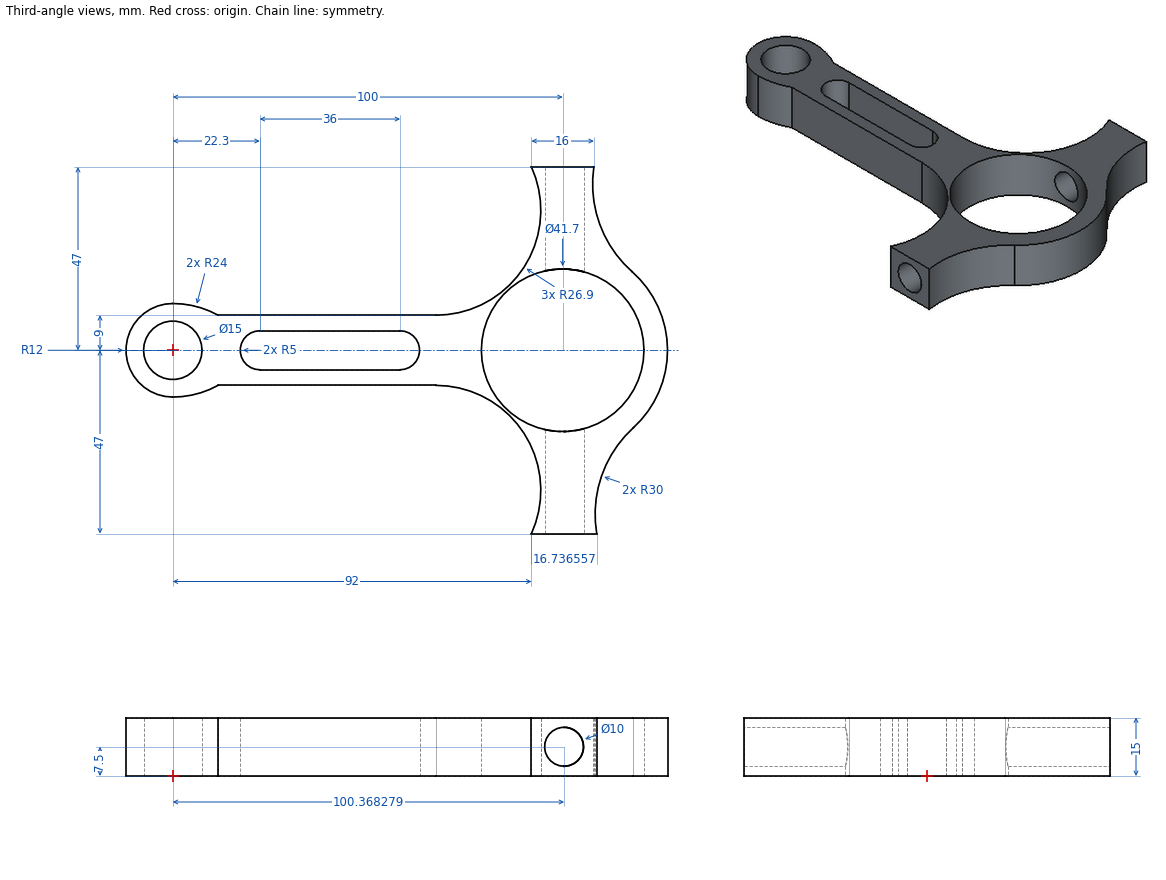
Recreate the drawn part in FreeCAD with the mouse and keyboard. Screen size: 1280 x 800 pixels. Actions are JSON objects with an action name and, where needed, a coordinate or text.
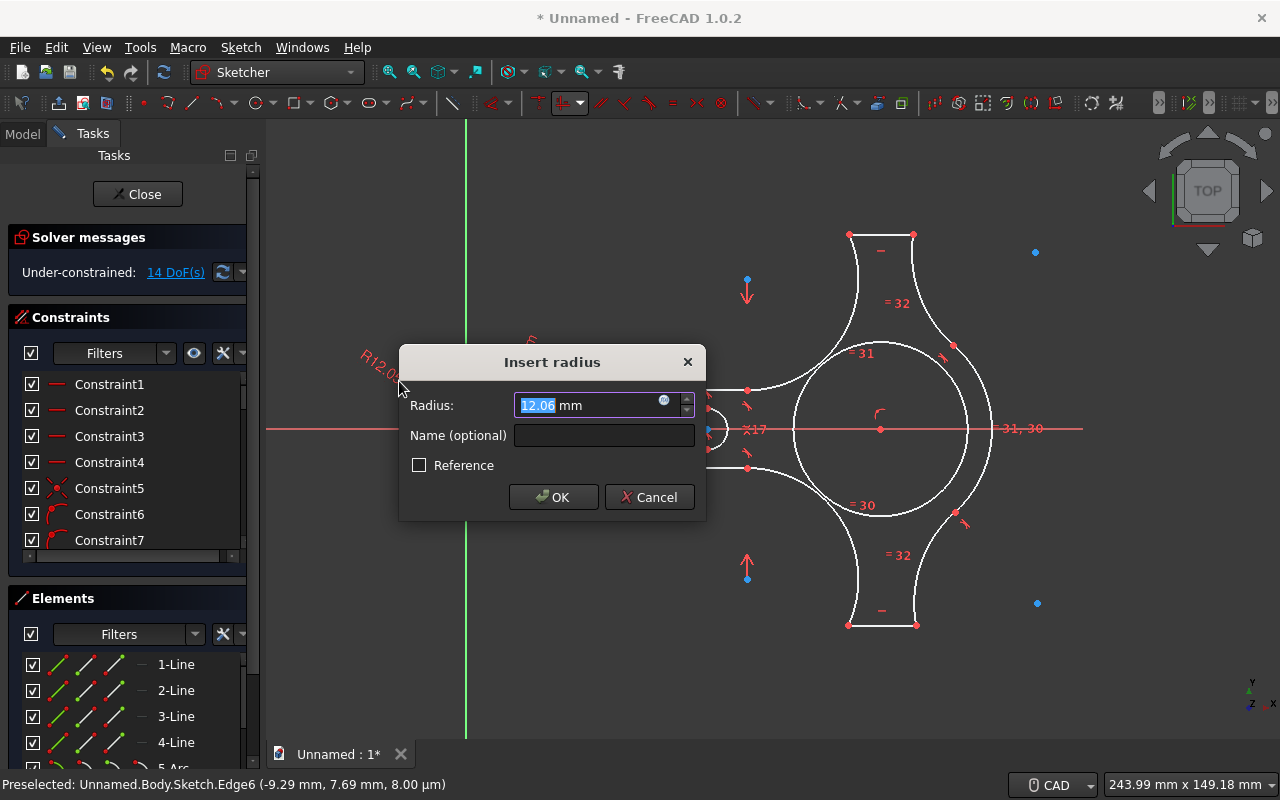
{"action": "type", "text": "12"}
{"action": "key", "text": "Return"}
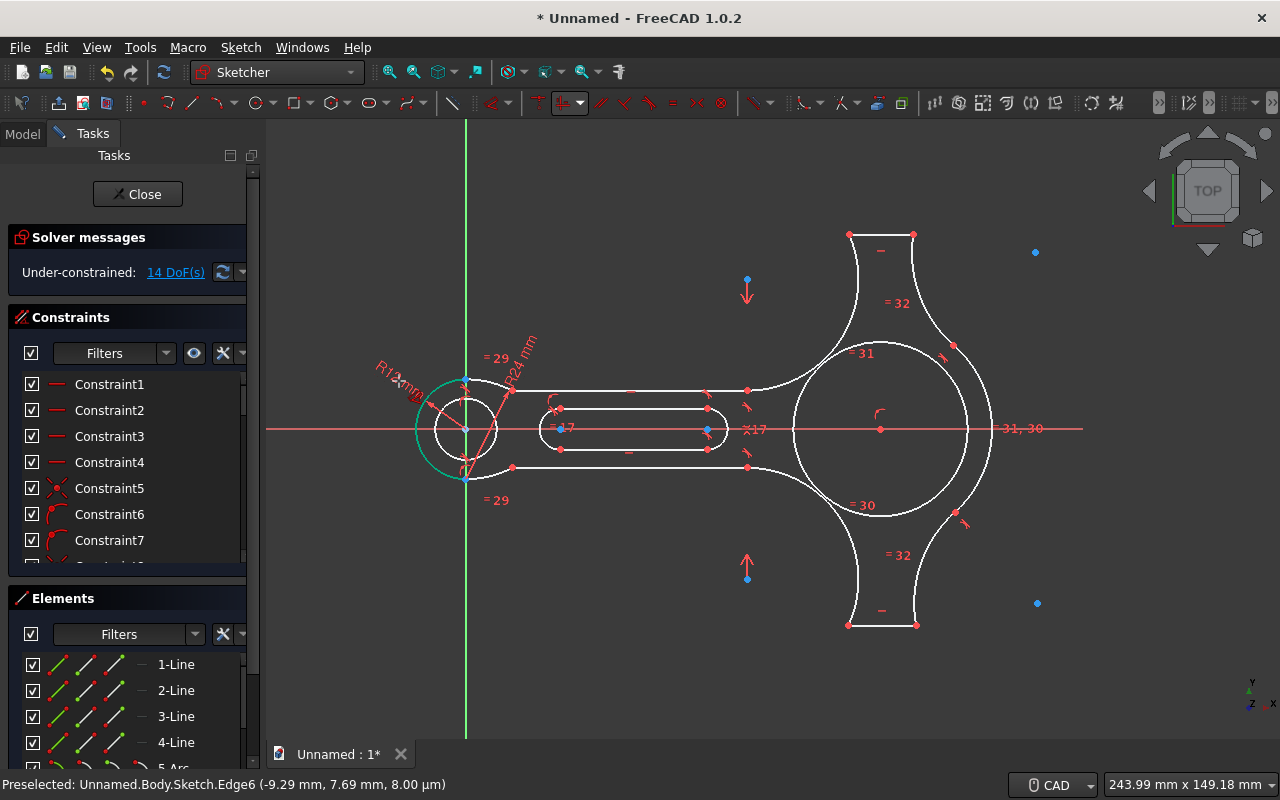
{"action": "left_click", "coordinate": [857, 560]}
{"action": "left_click", "coordinate": [889, 554]}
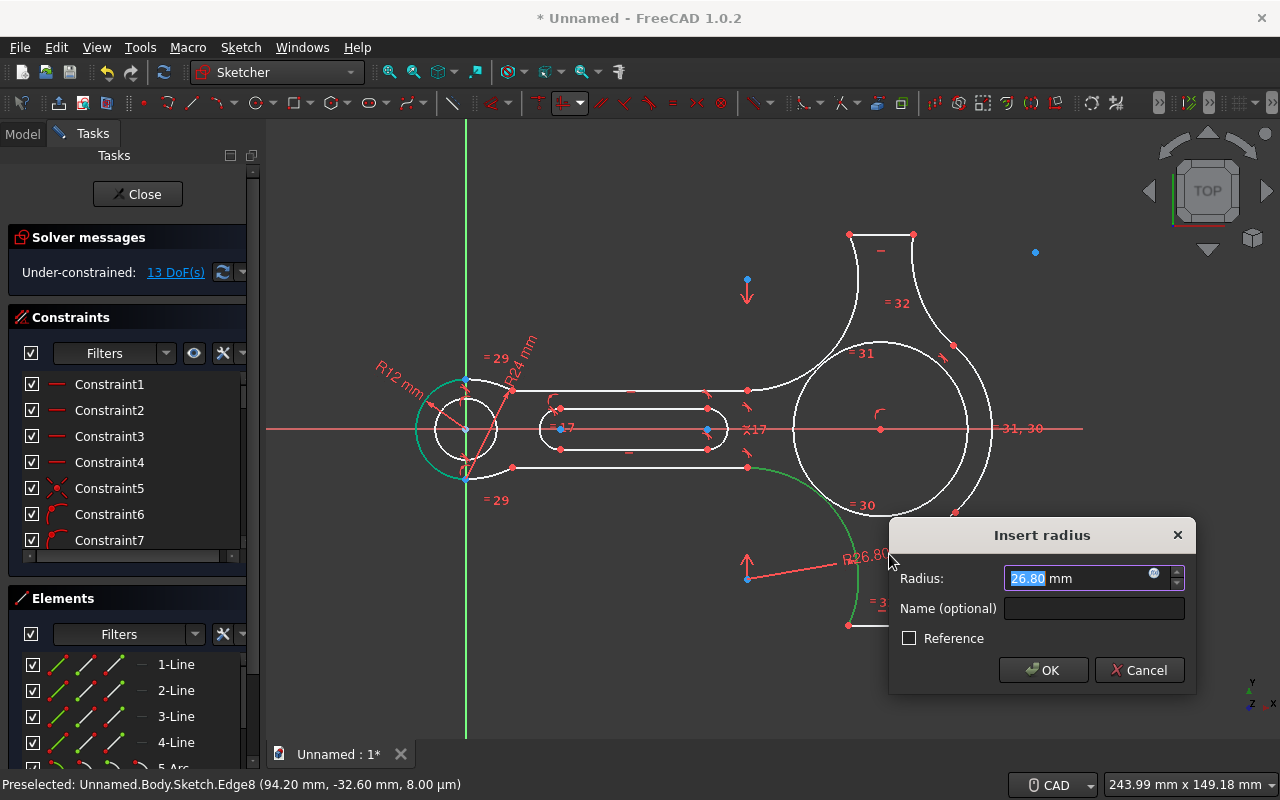
{"action": "type", "text": "26.9"}
{"action": "key", "text": "Return"}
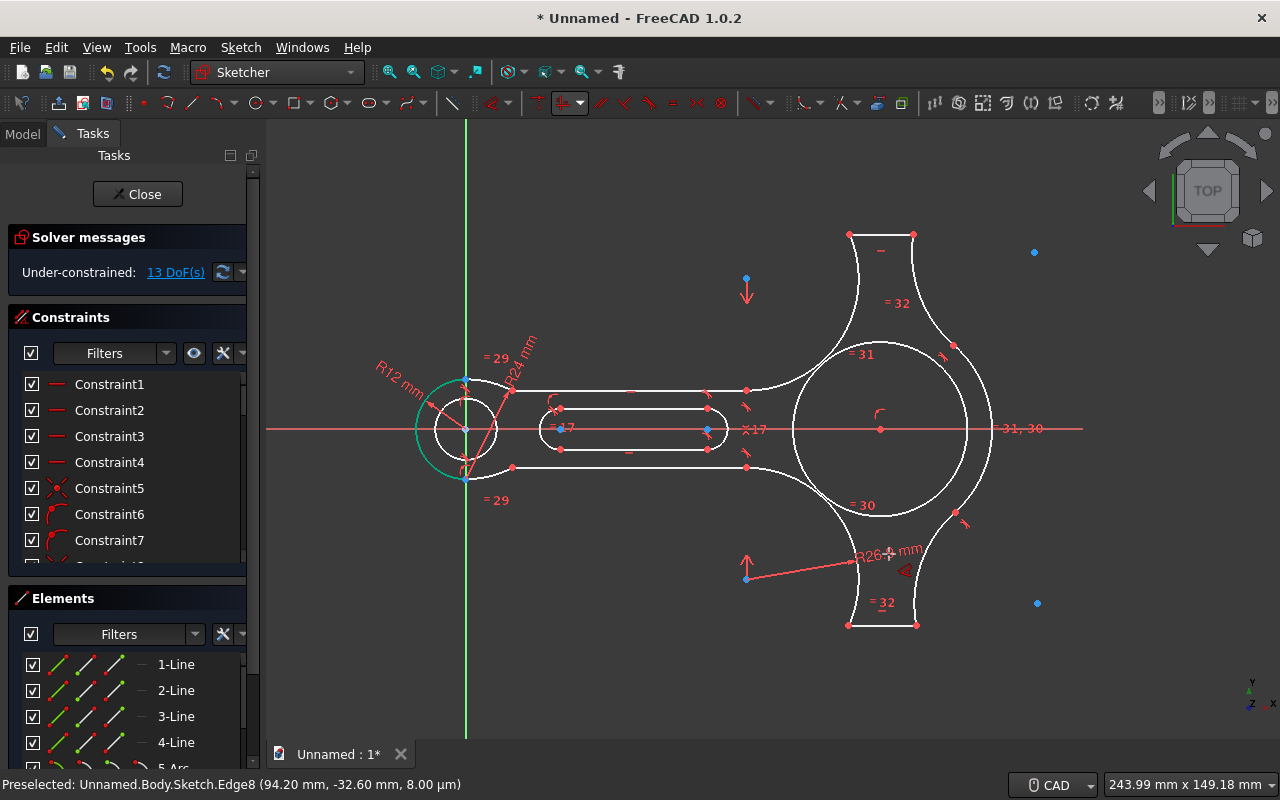
{"action": "left_click", "coordinate": [931, 541]}
{"action": "left_click", "coordinate": [882, 599]}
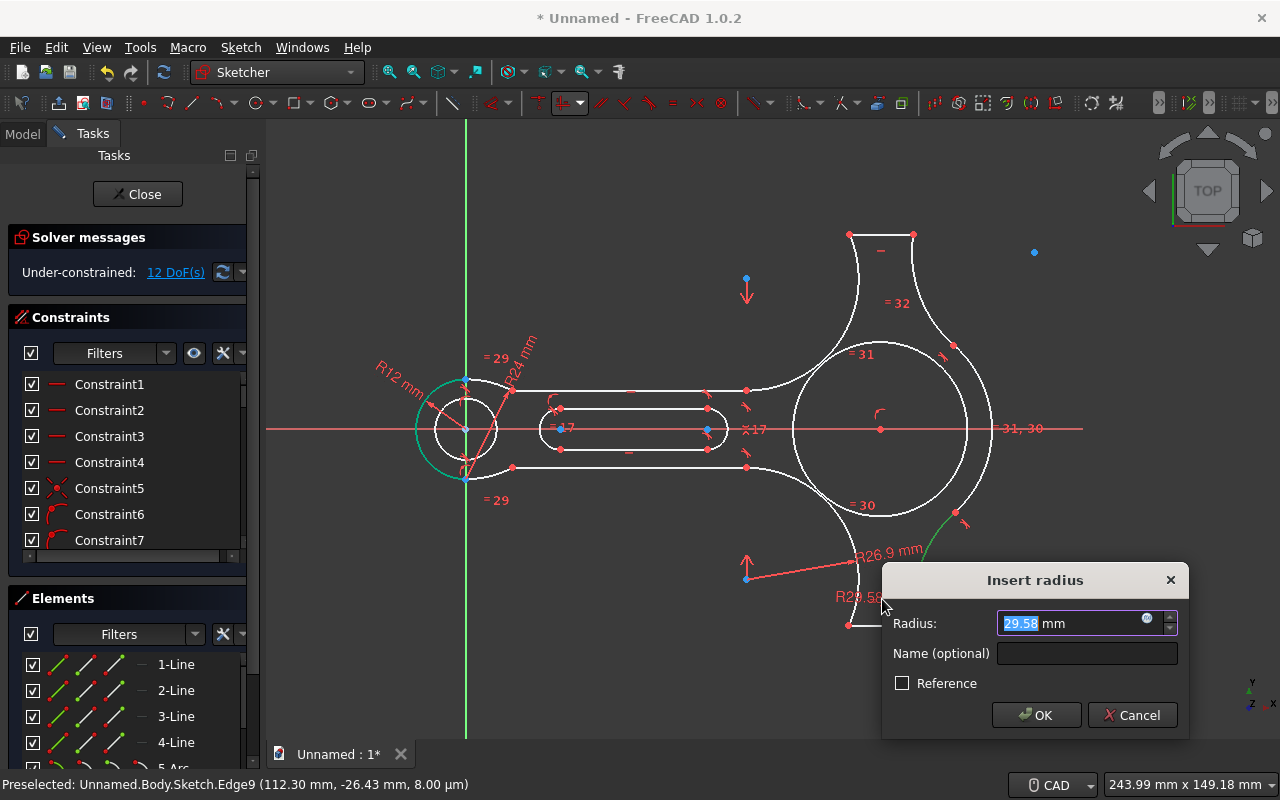
{"action": "type", "text": "30"}
{"action": "key", "text": "Return"}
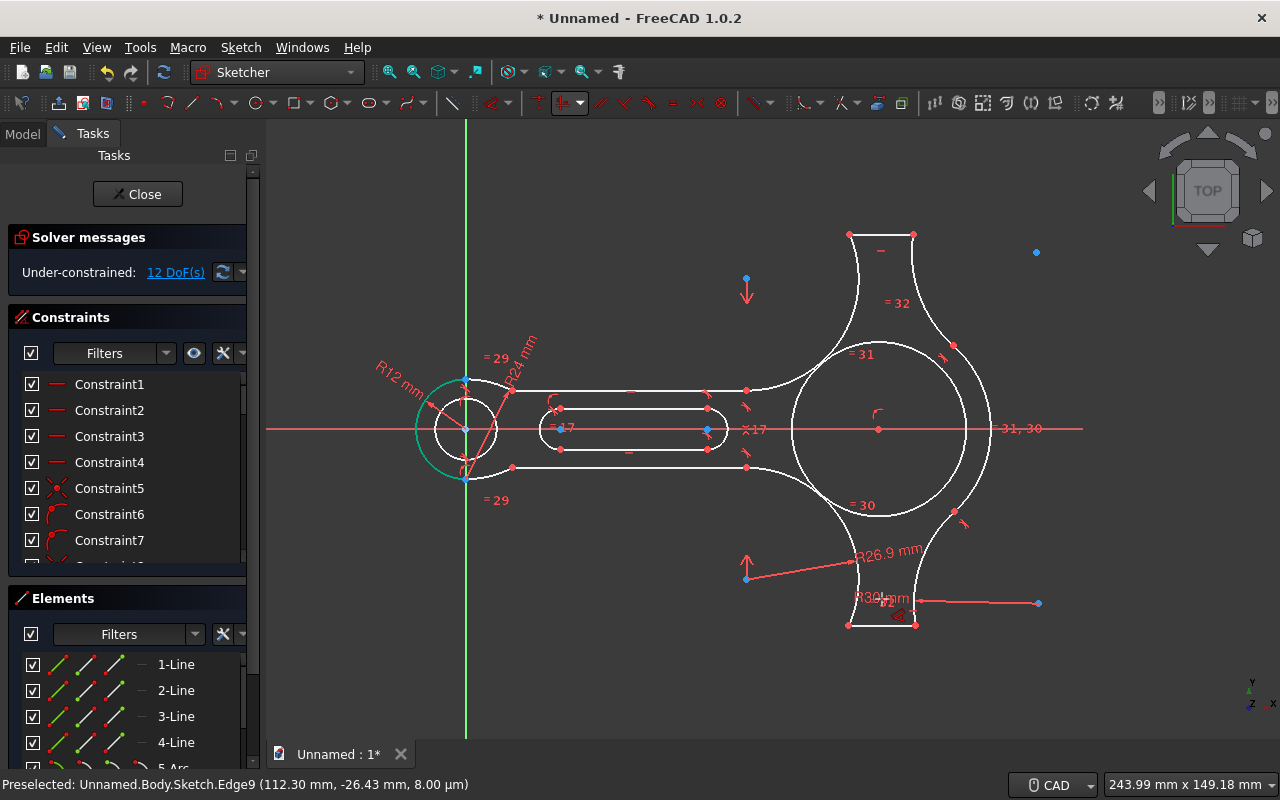
{"action": "scroll", "coordinate": [544, 417], "scroll_direction": "up", "scroll_amount": 4}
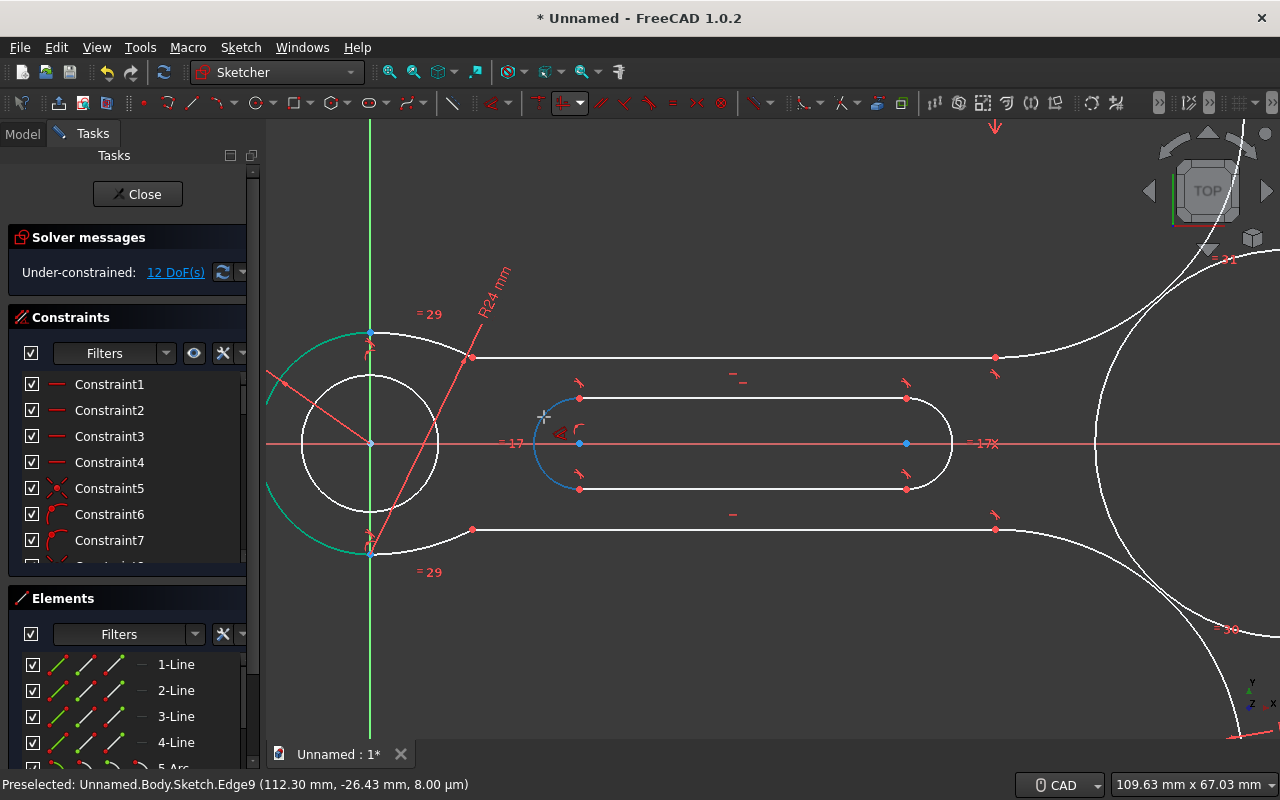
{"action": "left_click", "coordinate": [543, 417]}
{"action": "left_click", "coordinate": [517, 398]}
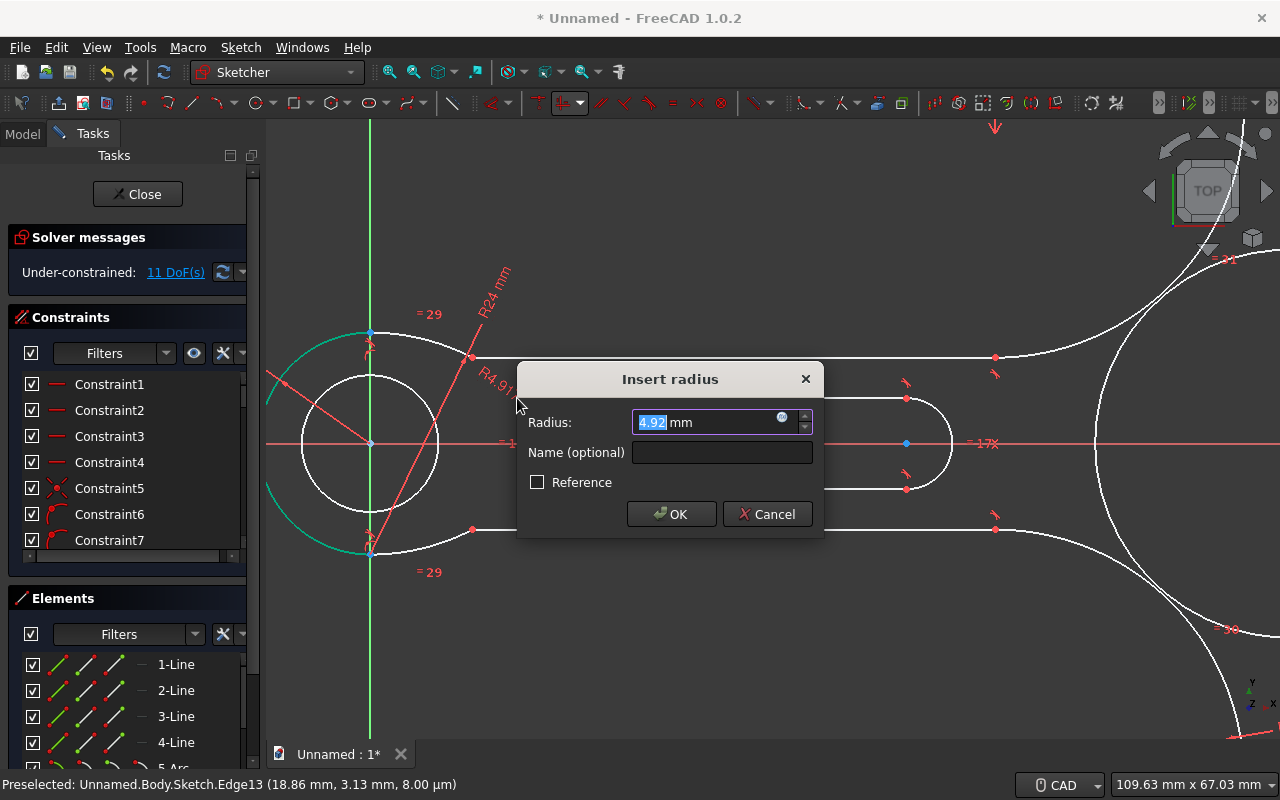
{"action": "type", "text": "5"}
{"action": "key", "text": "Return"}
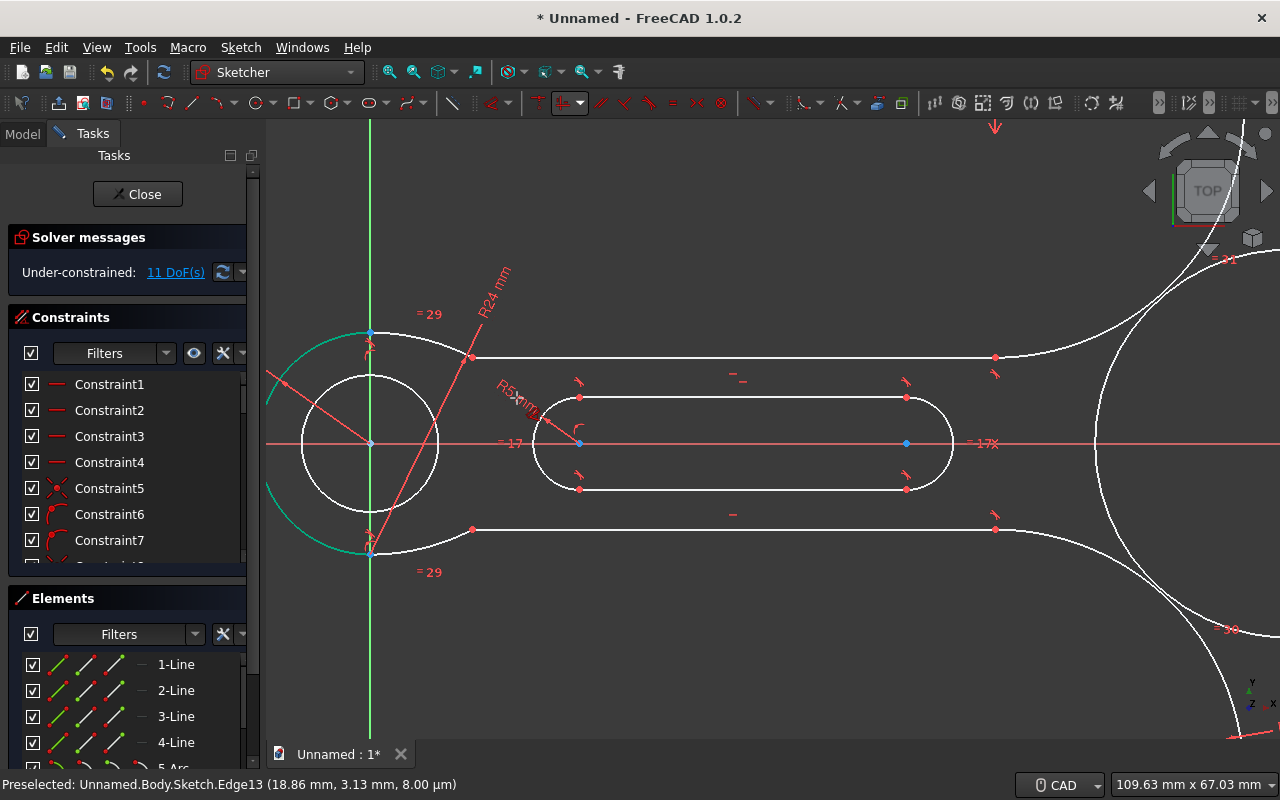
{"action": "left_click", "coordinate": [418, 395]}
{"action": "left_click", "coordinate": [440, 372]}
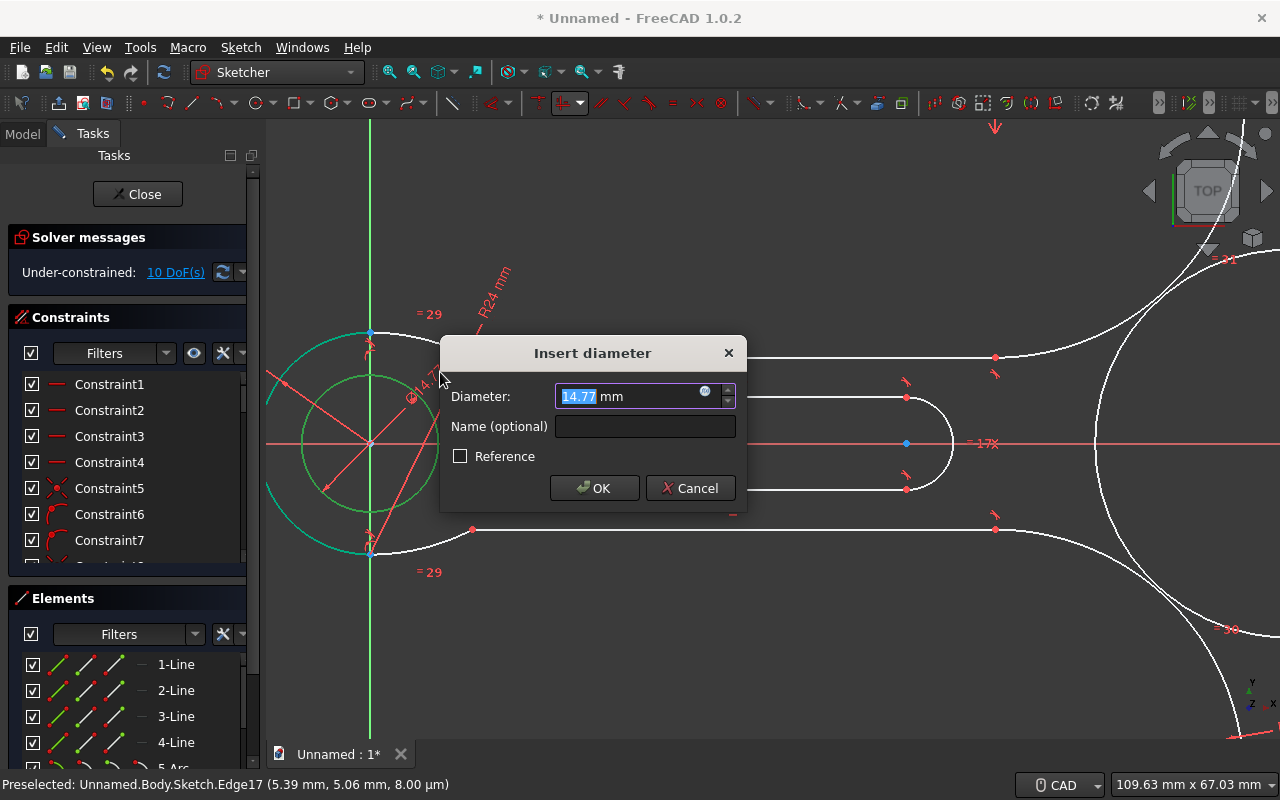
{"action": "type", "text": "15"}
{"action": "key", "text": "Return"}